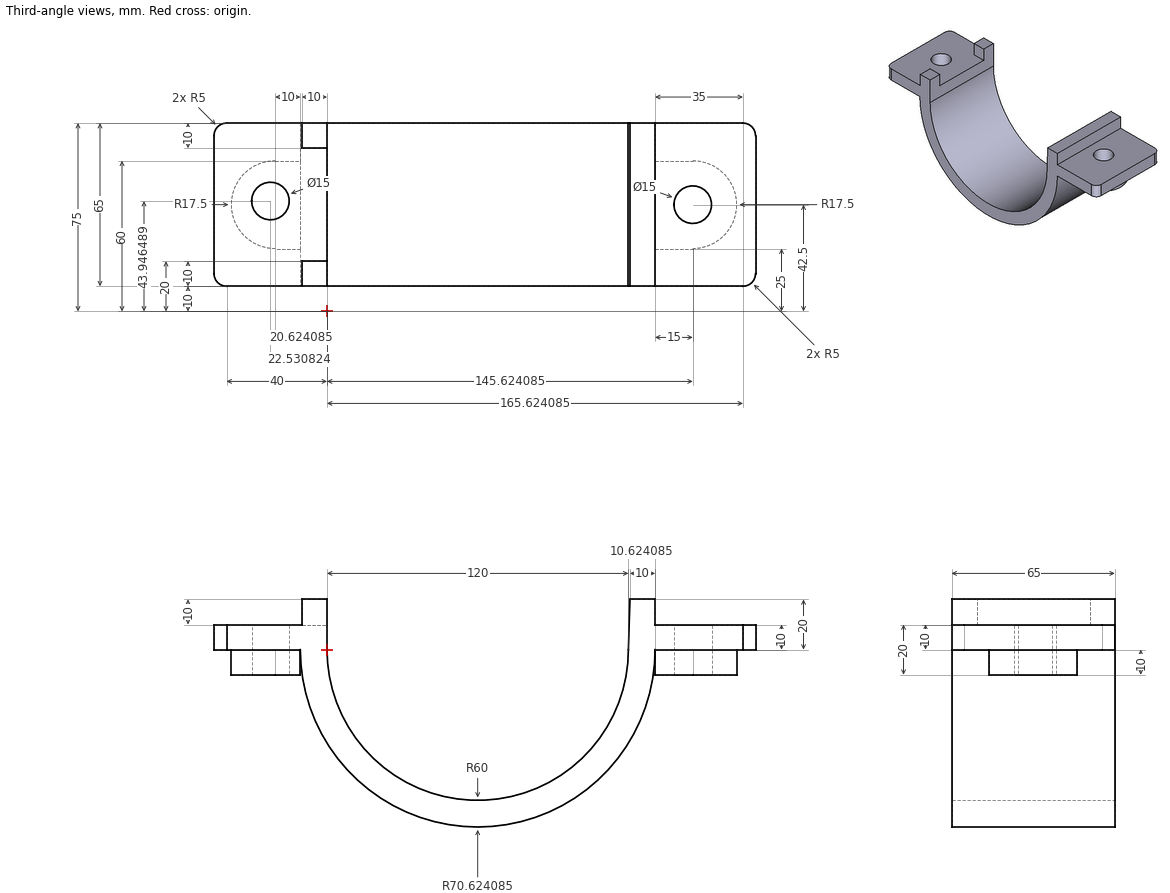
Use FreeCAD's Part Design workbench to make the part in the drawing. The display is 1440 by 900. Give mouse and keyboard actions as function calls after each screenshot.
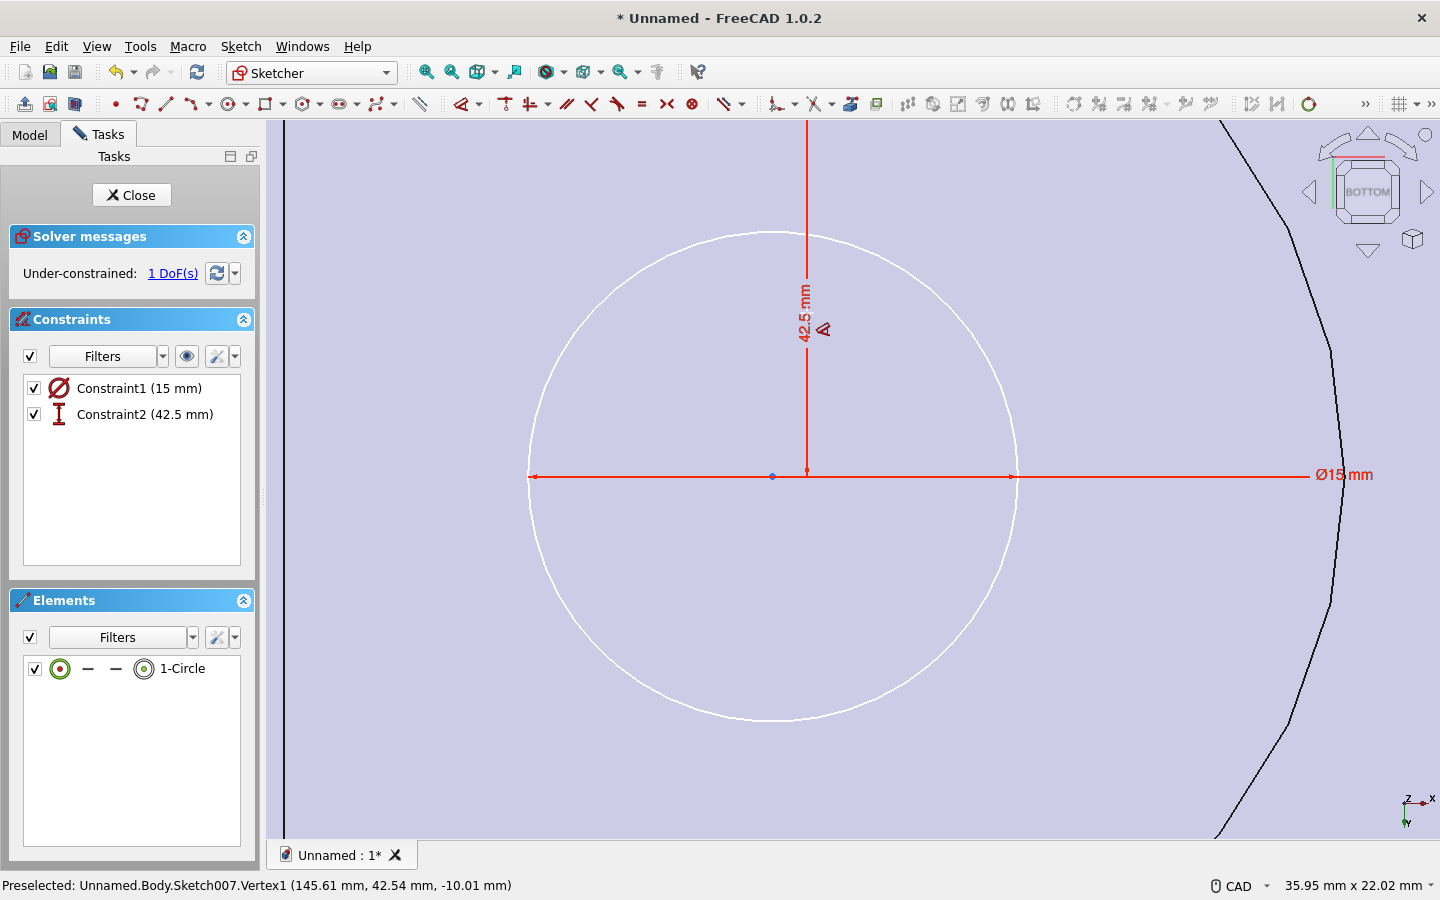
click(773, 477)
click(423, 511)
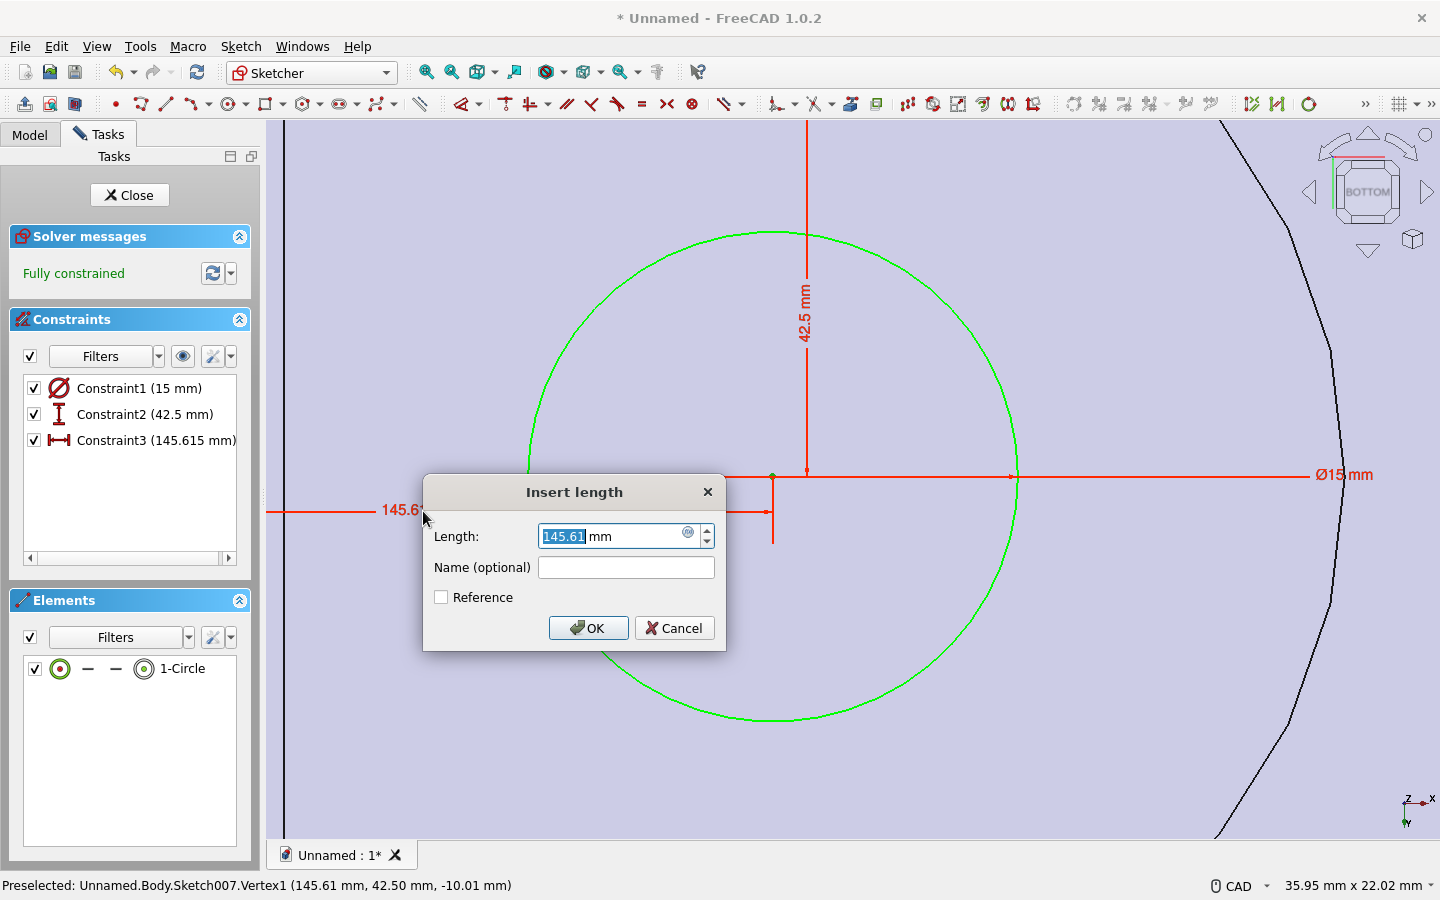
text(145.624085)
key(Return)
key(Escape)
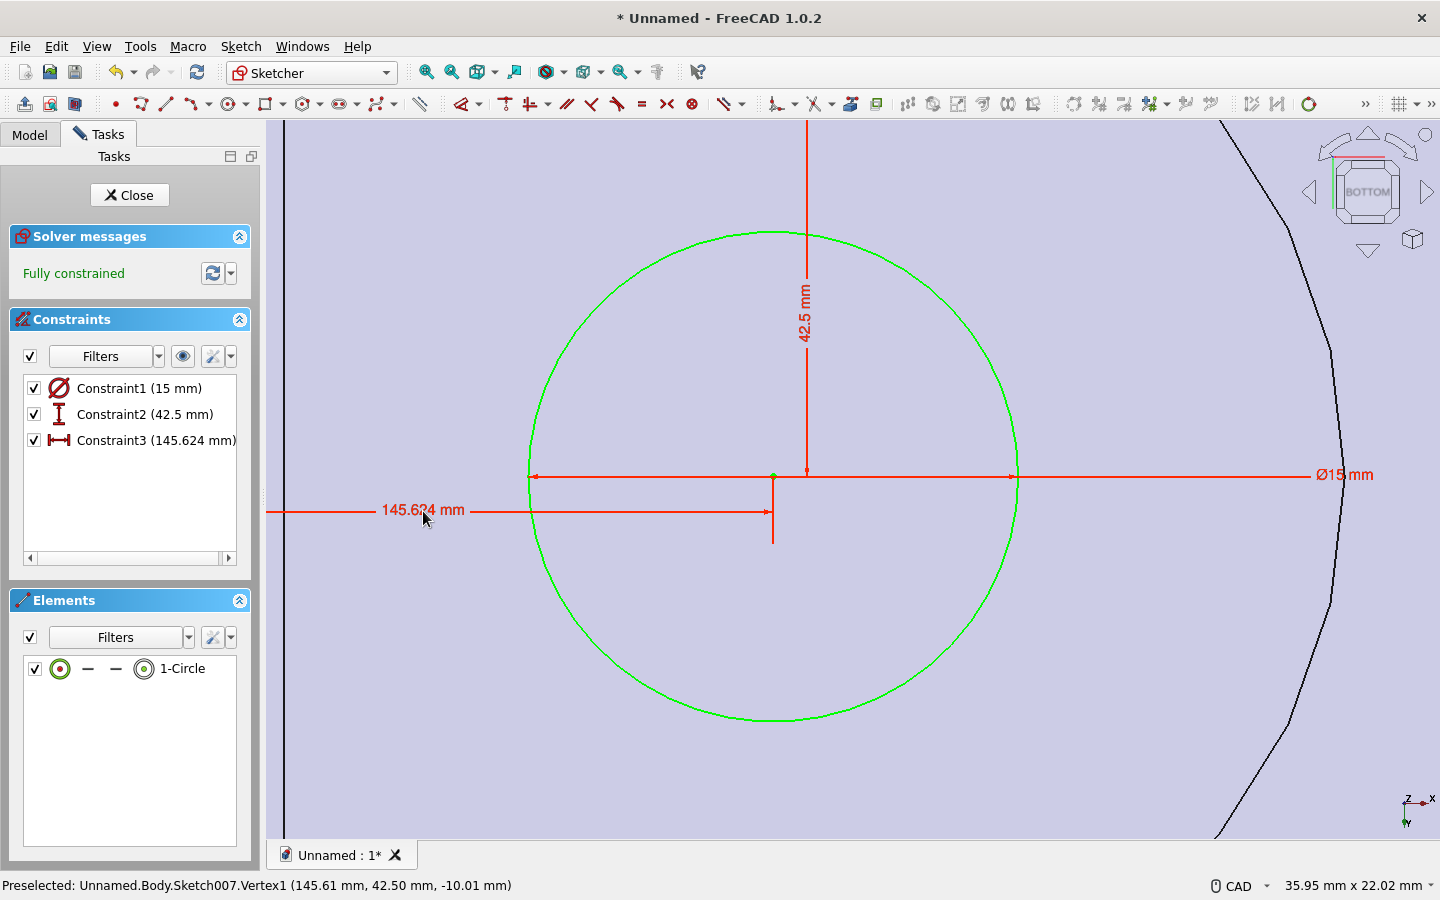
click(130, 195)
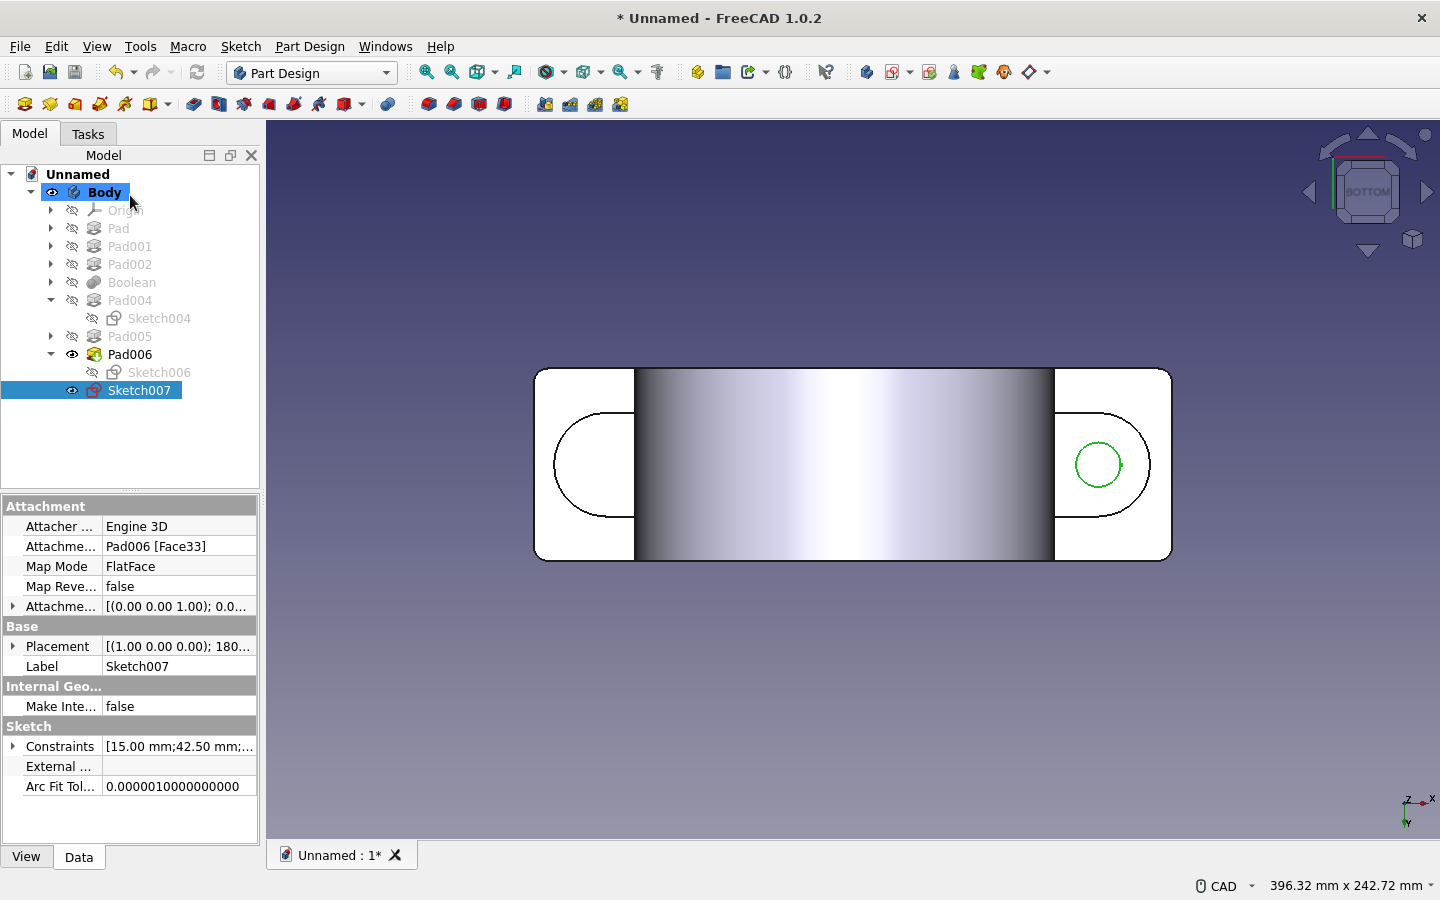
click(194, 104)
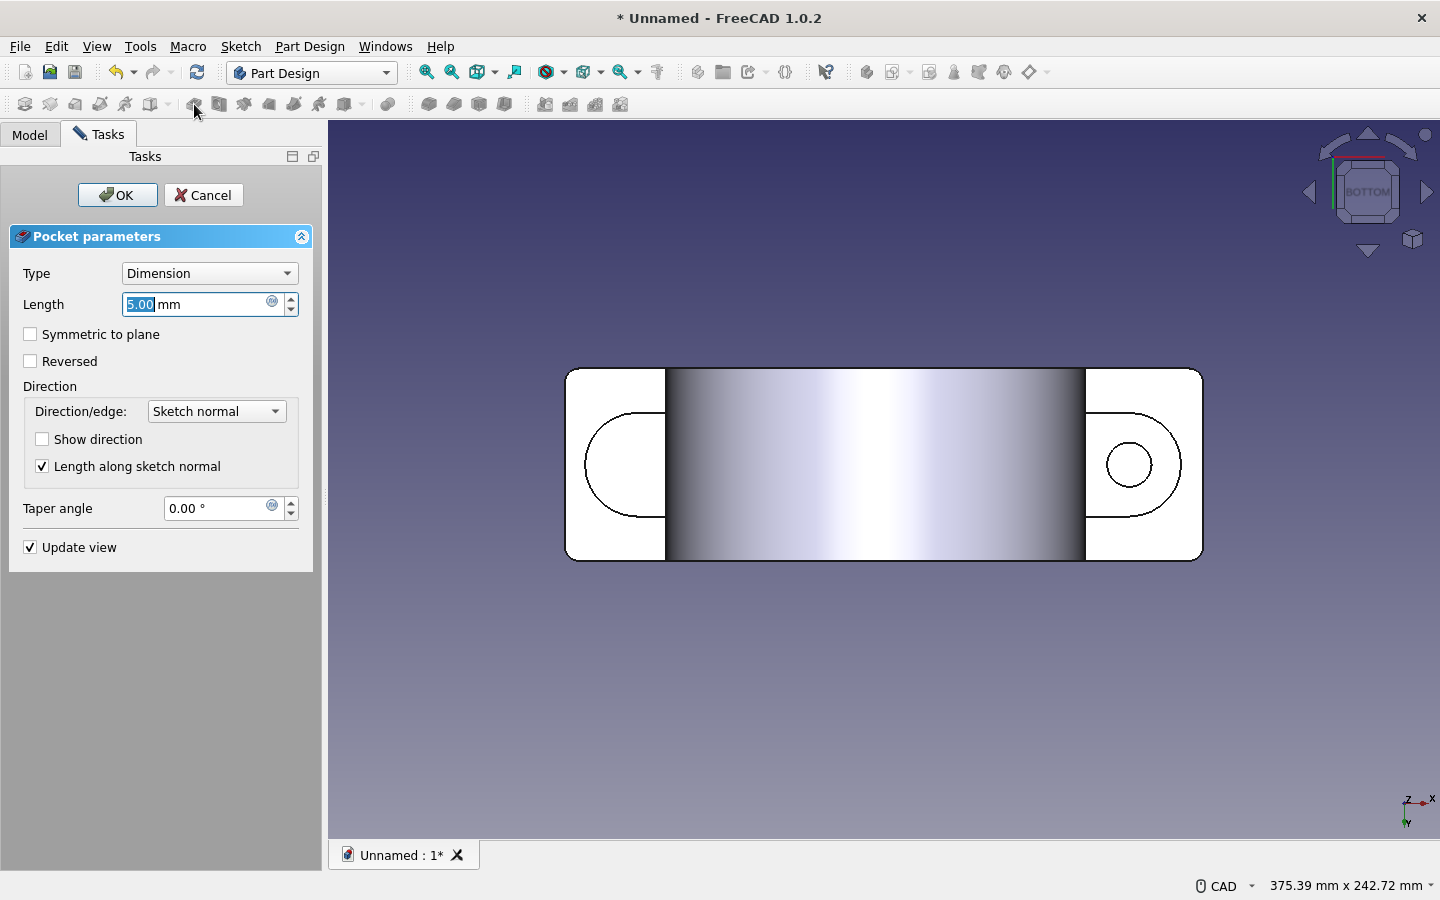
text(20)
key(Tab)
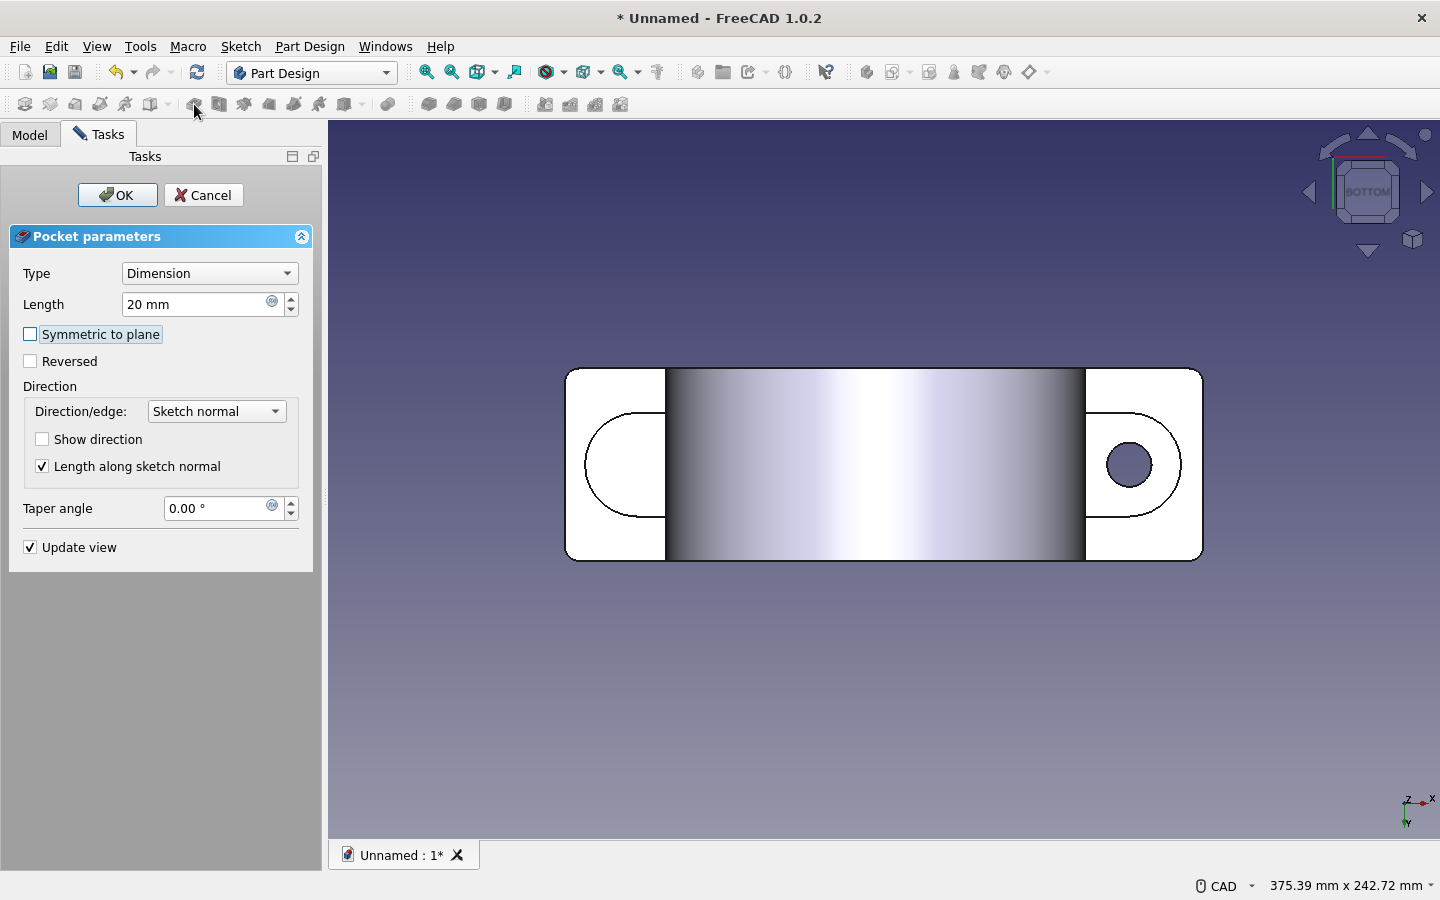
click(118, 195)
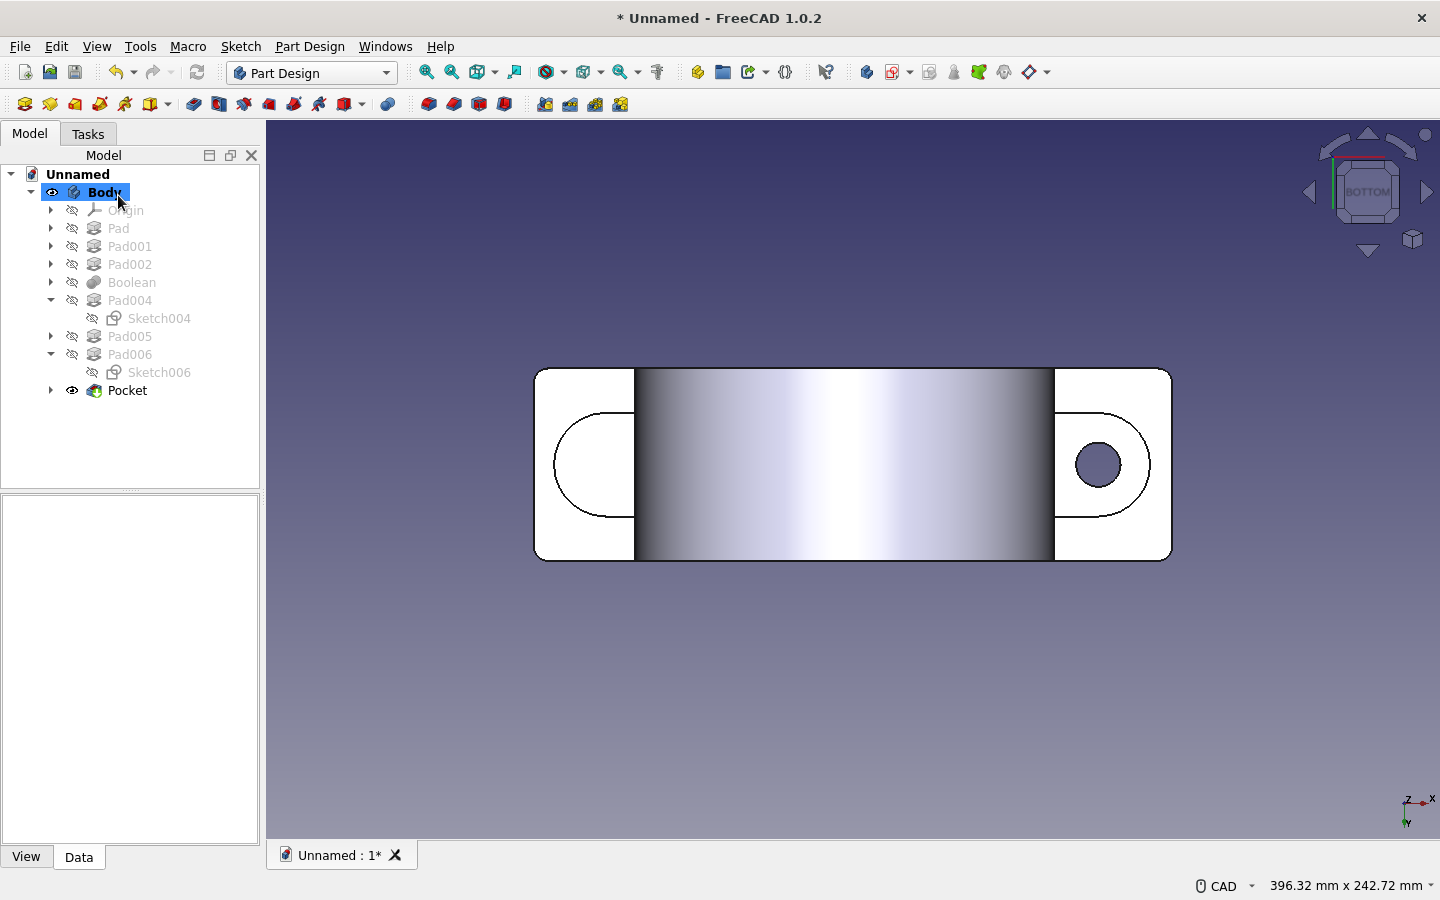
click(595, 464)